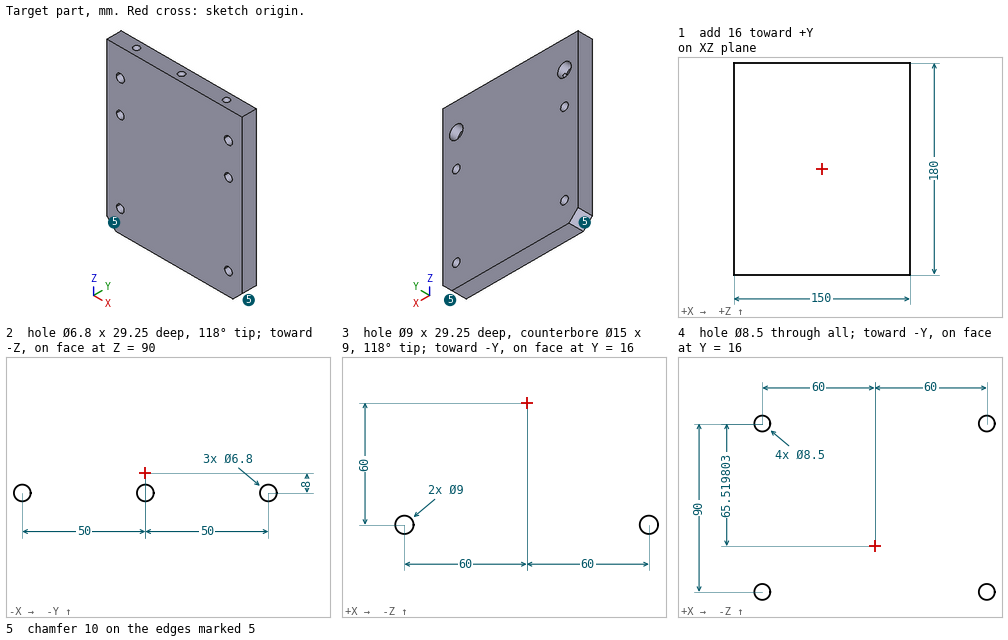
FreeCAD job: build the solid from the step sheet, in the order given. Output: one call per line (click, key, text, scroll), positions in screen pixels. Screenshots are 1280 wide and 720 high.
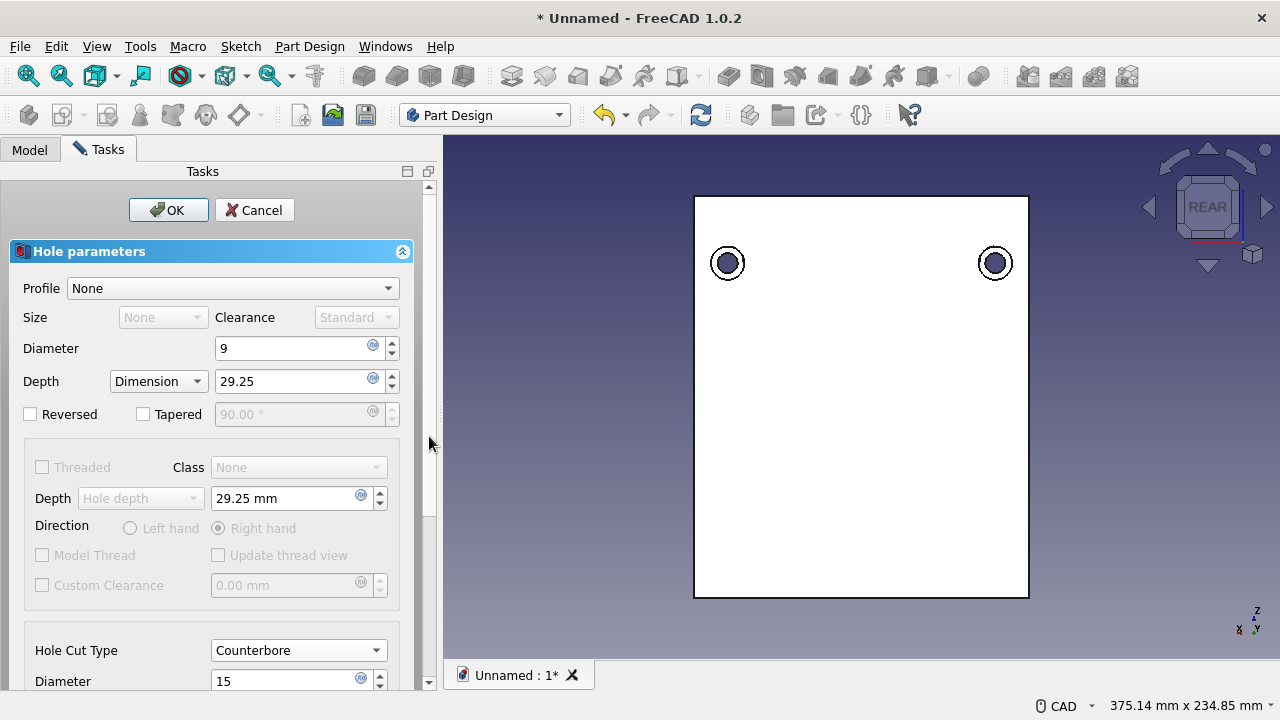
click(169, 210)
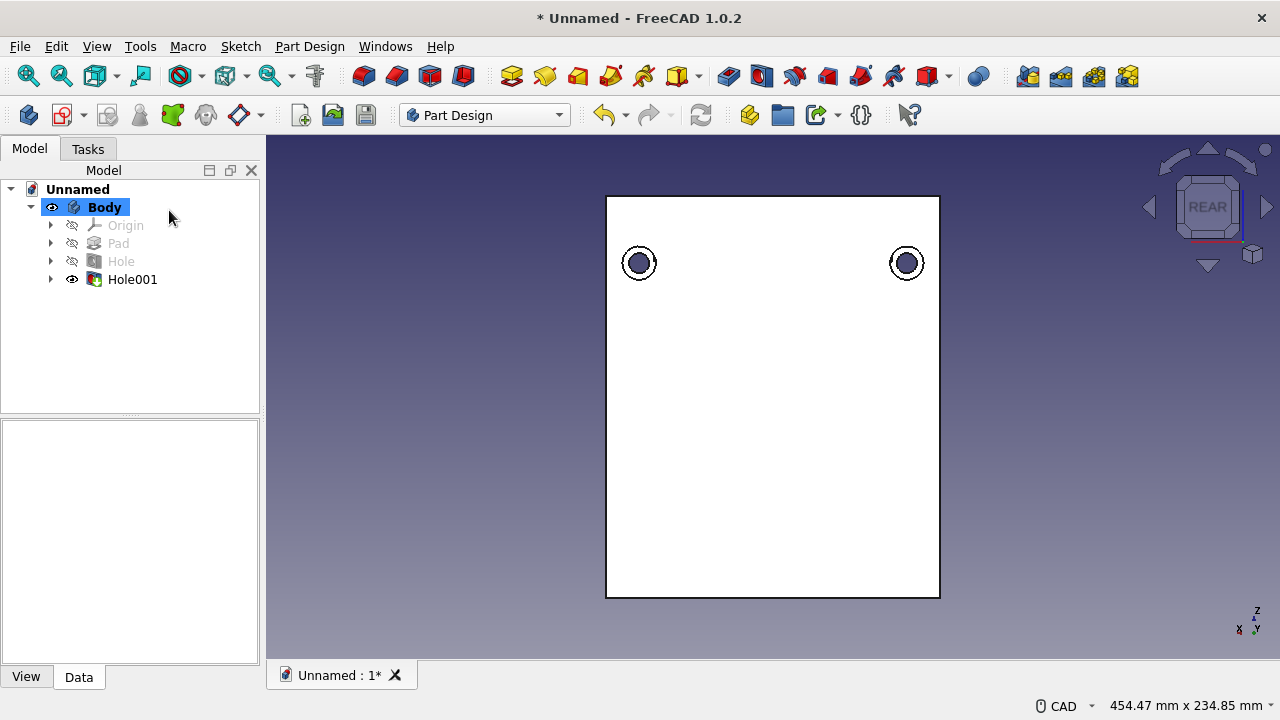
click(773, 396)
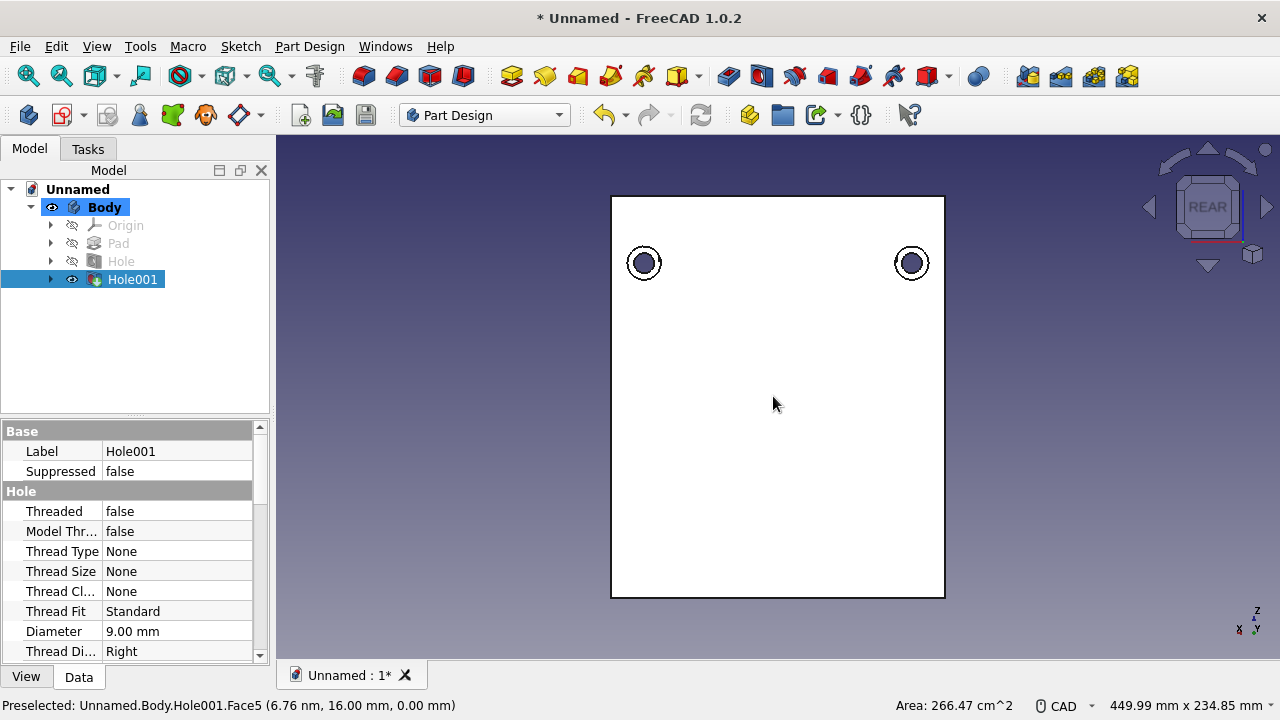
click(62, 116)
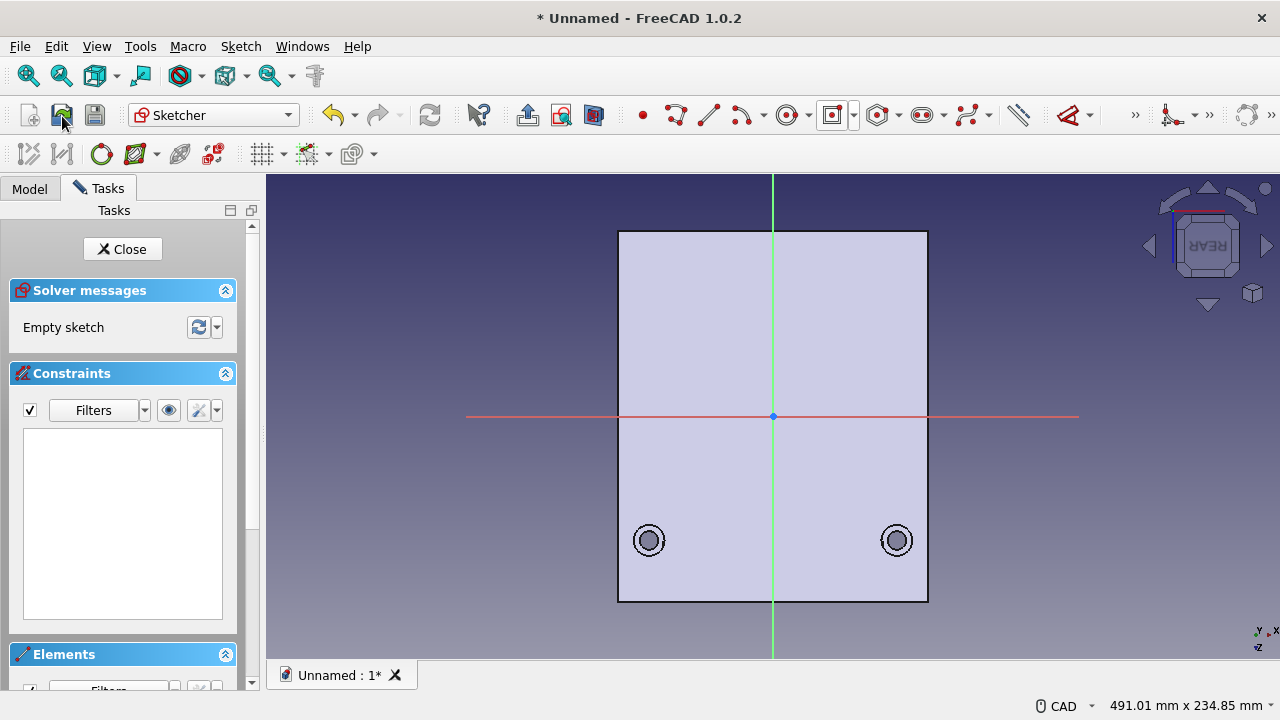
scroll(912, 288, up, 2)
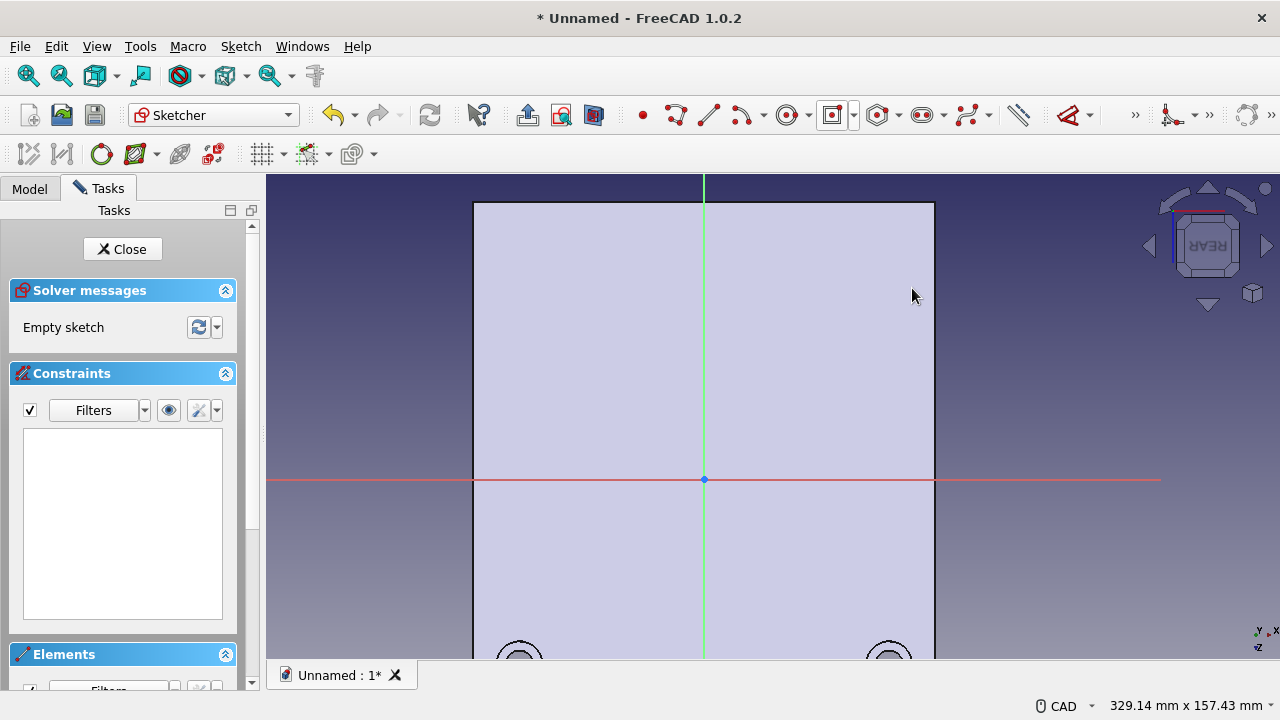
click(786, 116)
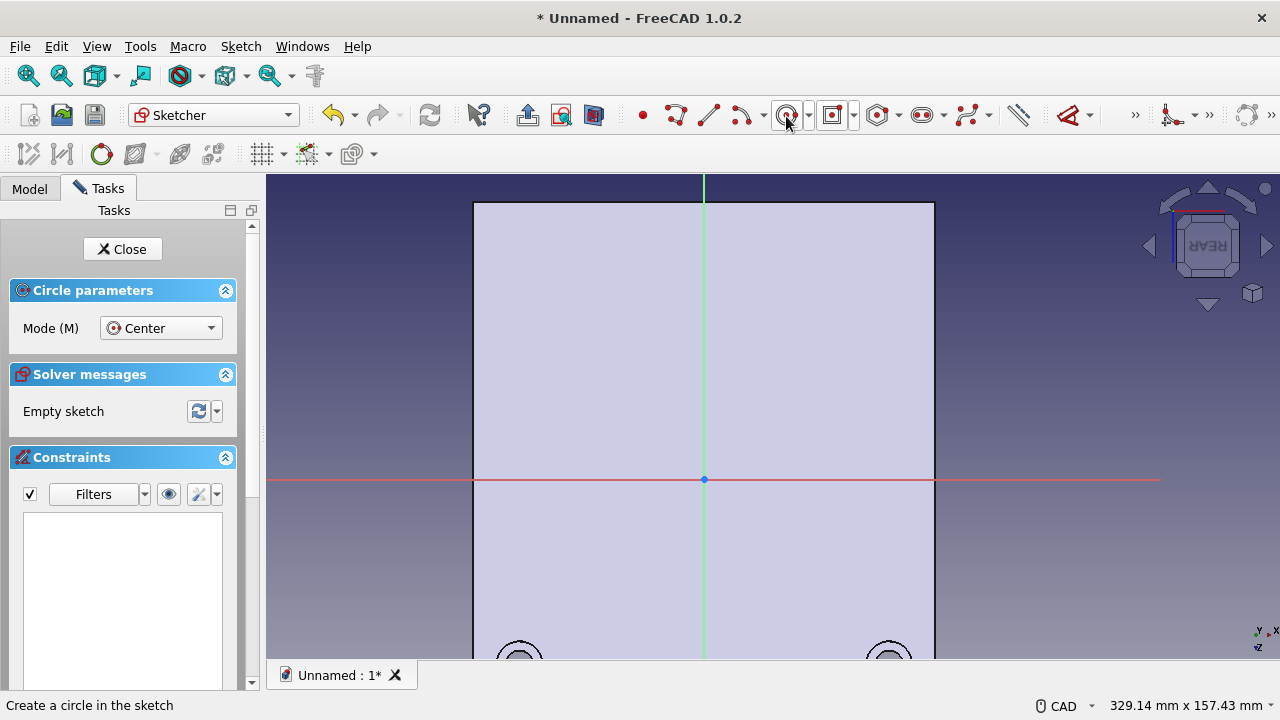
scroll(519, 278, up, 3)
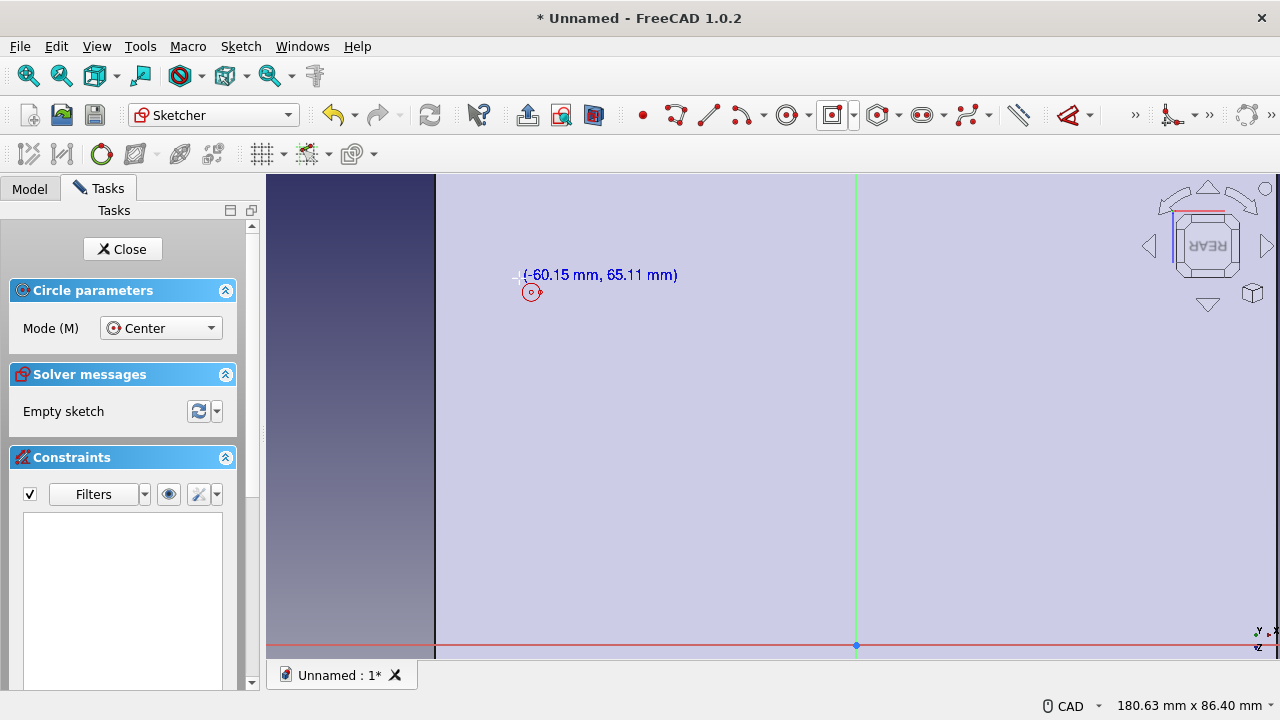
click(520, 277)
move(537, 260)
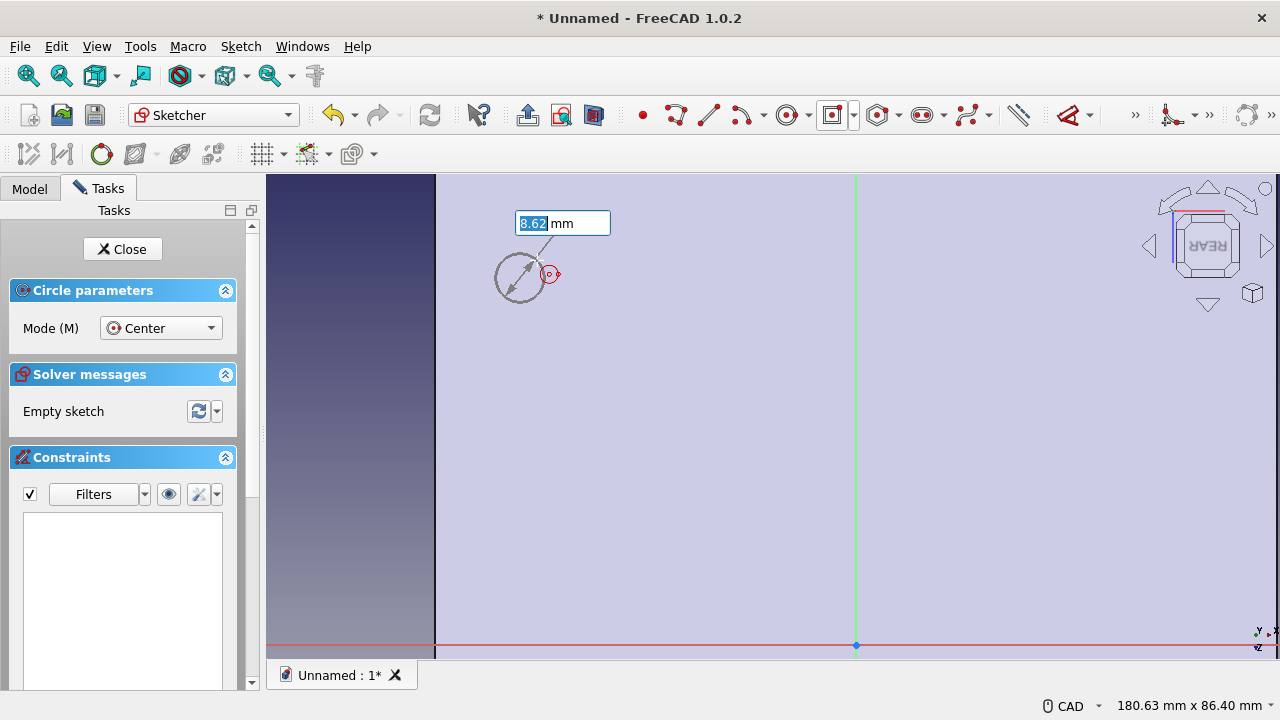
text(8.5)
key(Return)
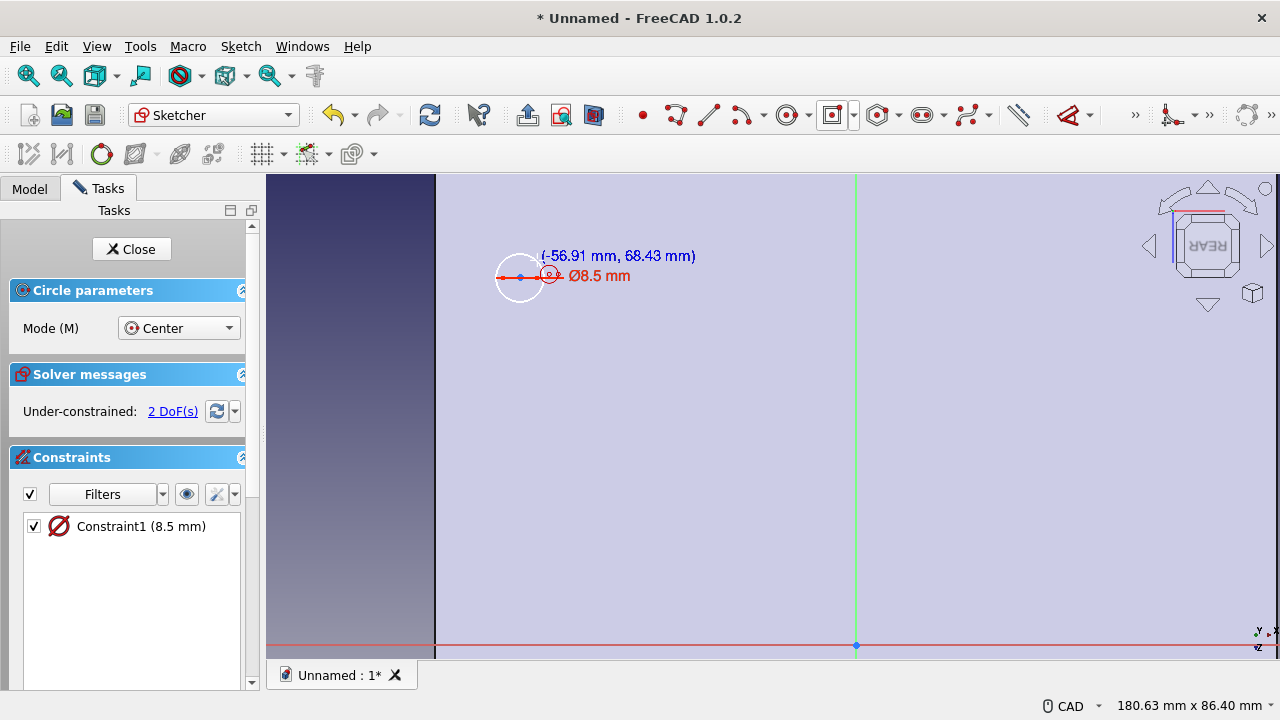
scroll(520, 279, down, 3)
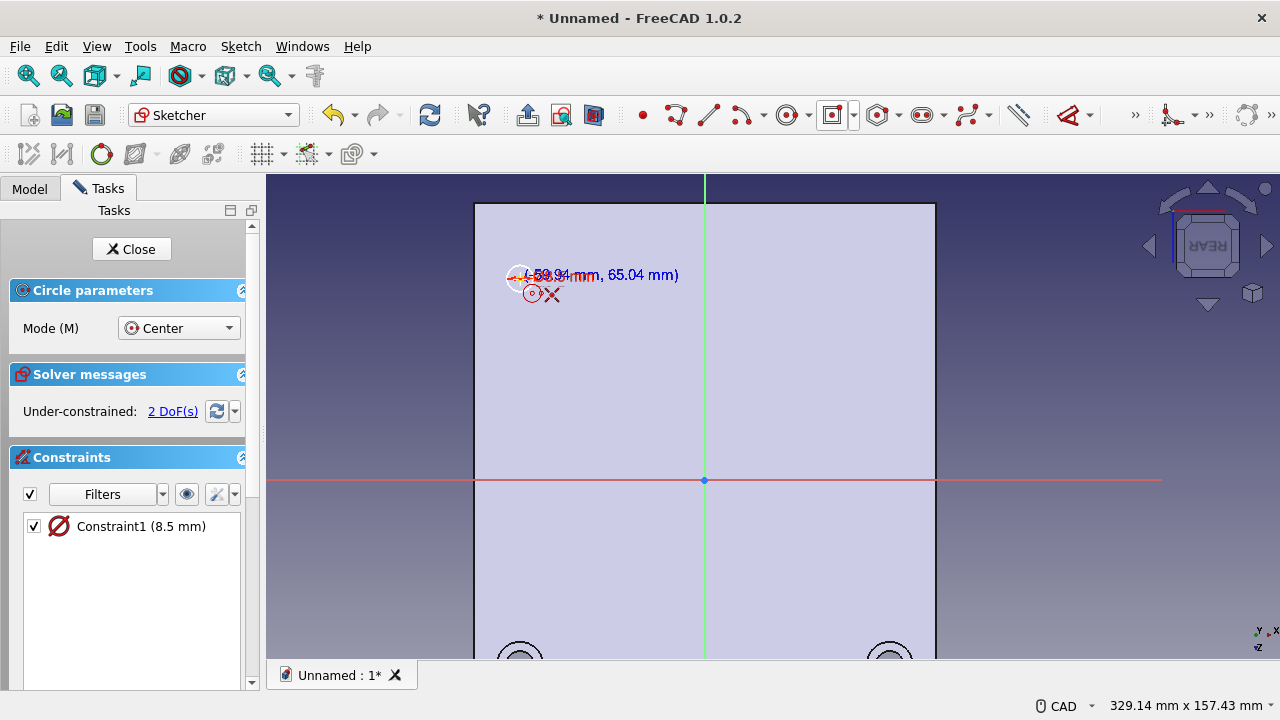
scroll(890, 278, up, 3)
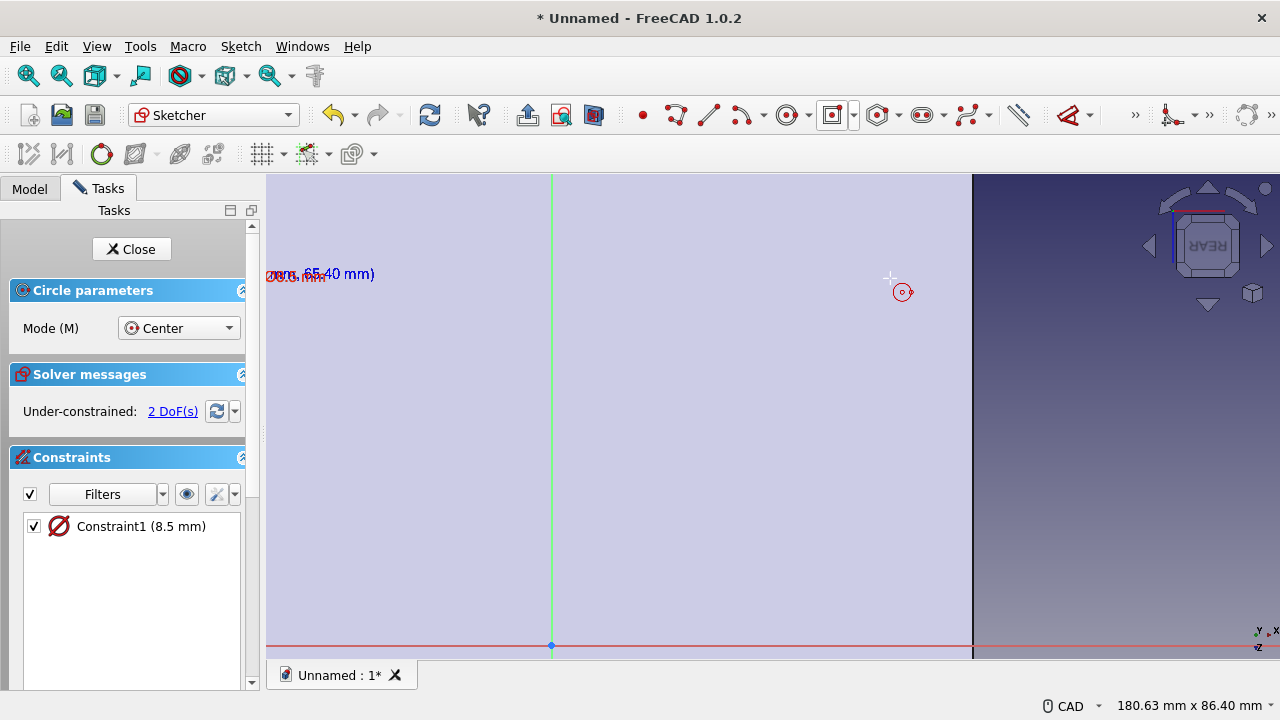
click(889, 278)
move(906, 261)